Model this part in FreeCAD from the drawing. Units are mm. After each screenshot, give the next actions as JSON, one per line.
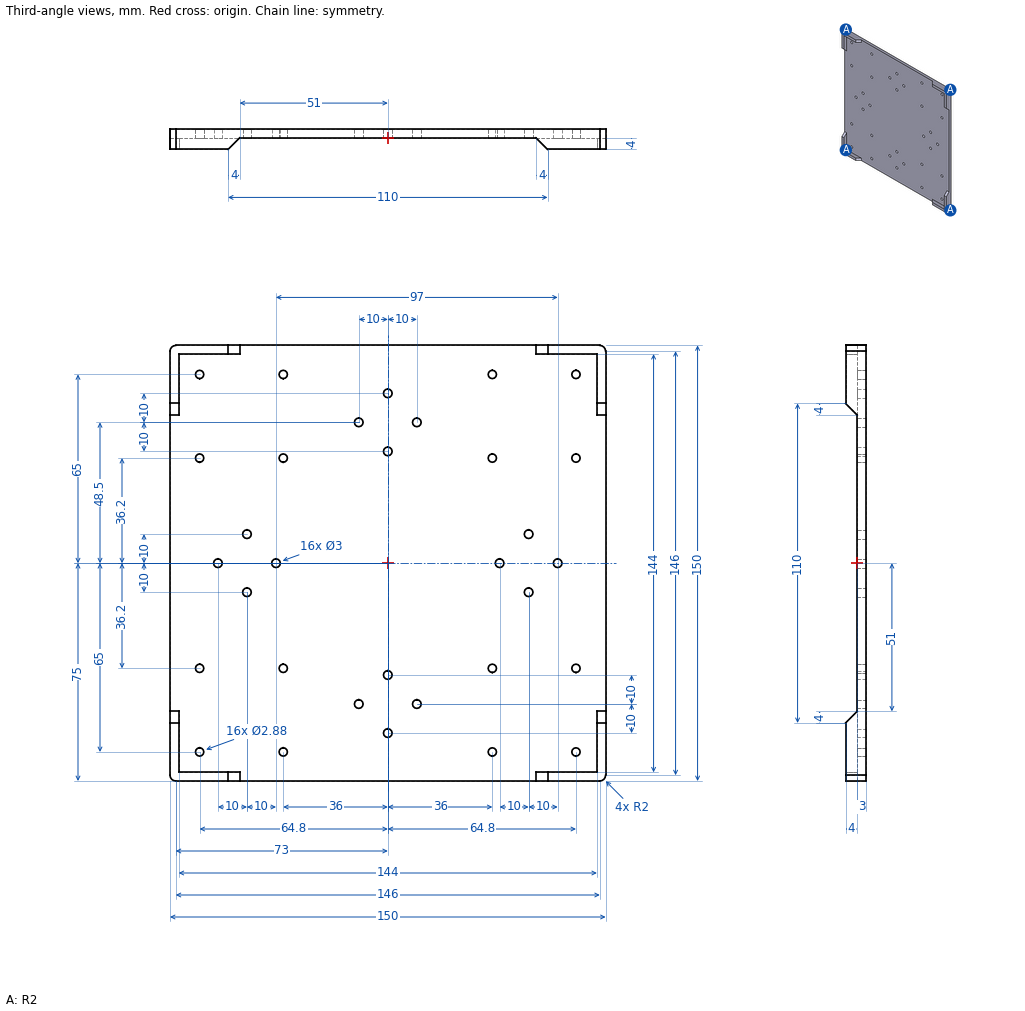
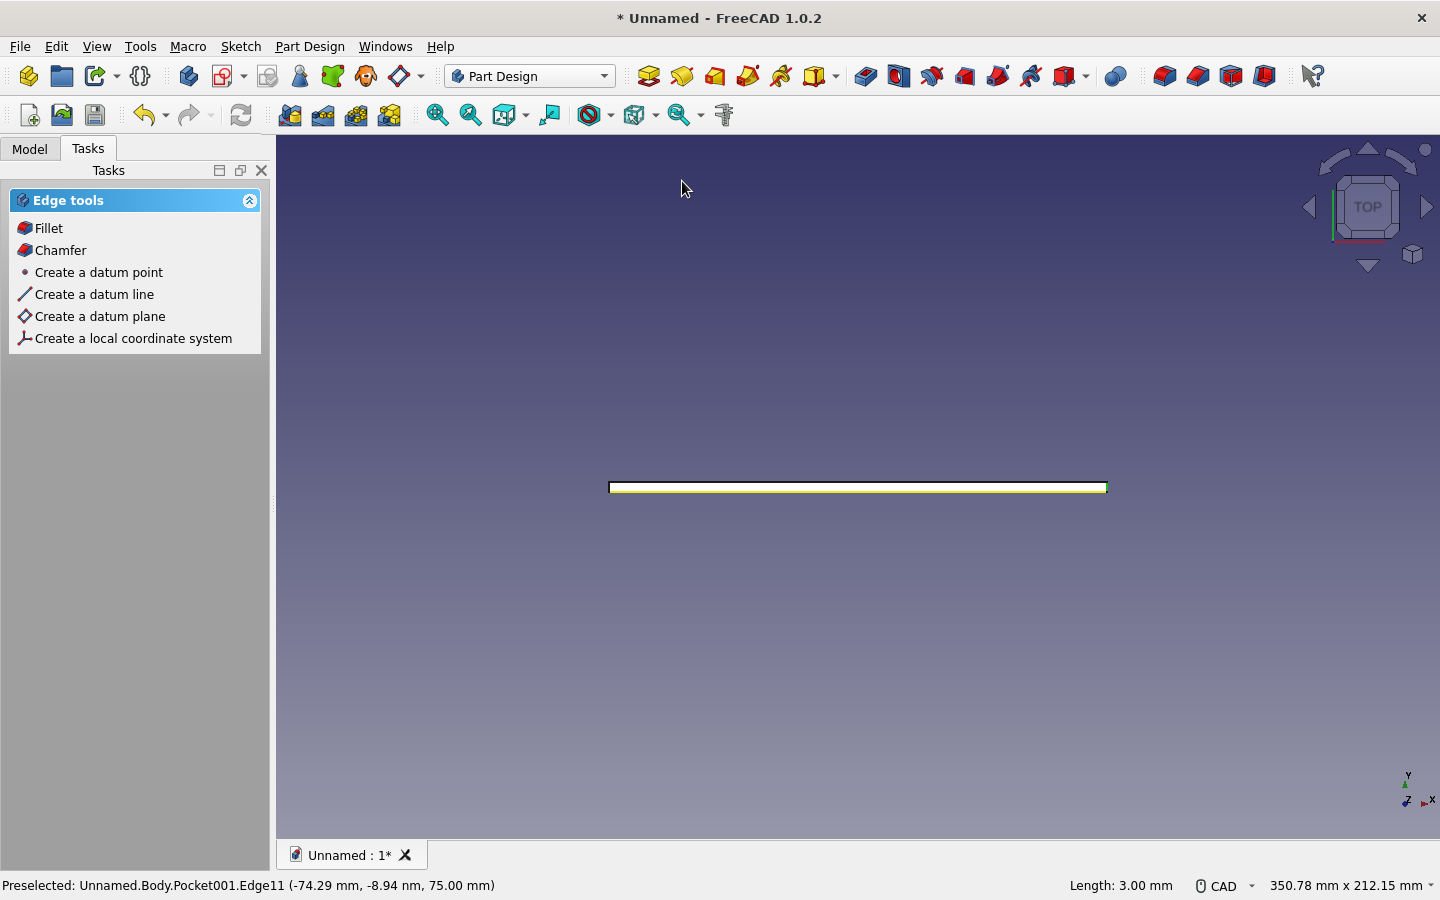
{"action": "left_click", "coordinate": [438, 116]}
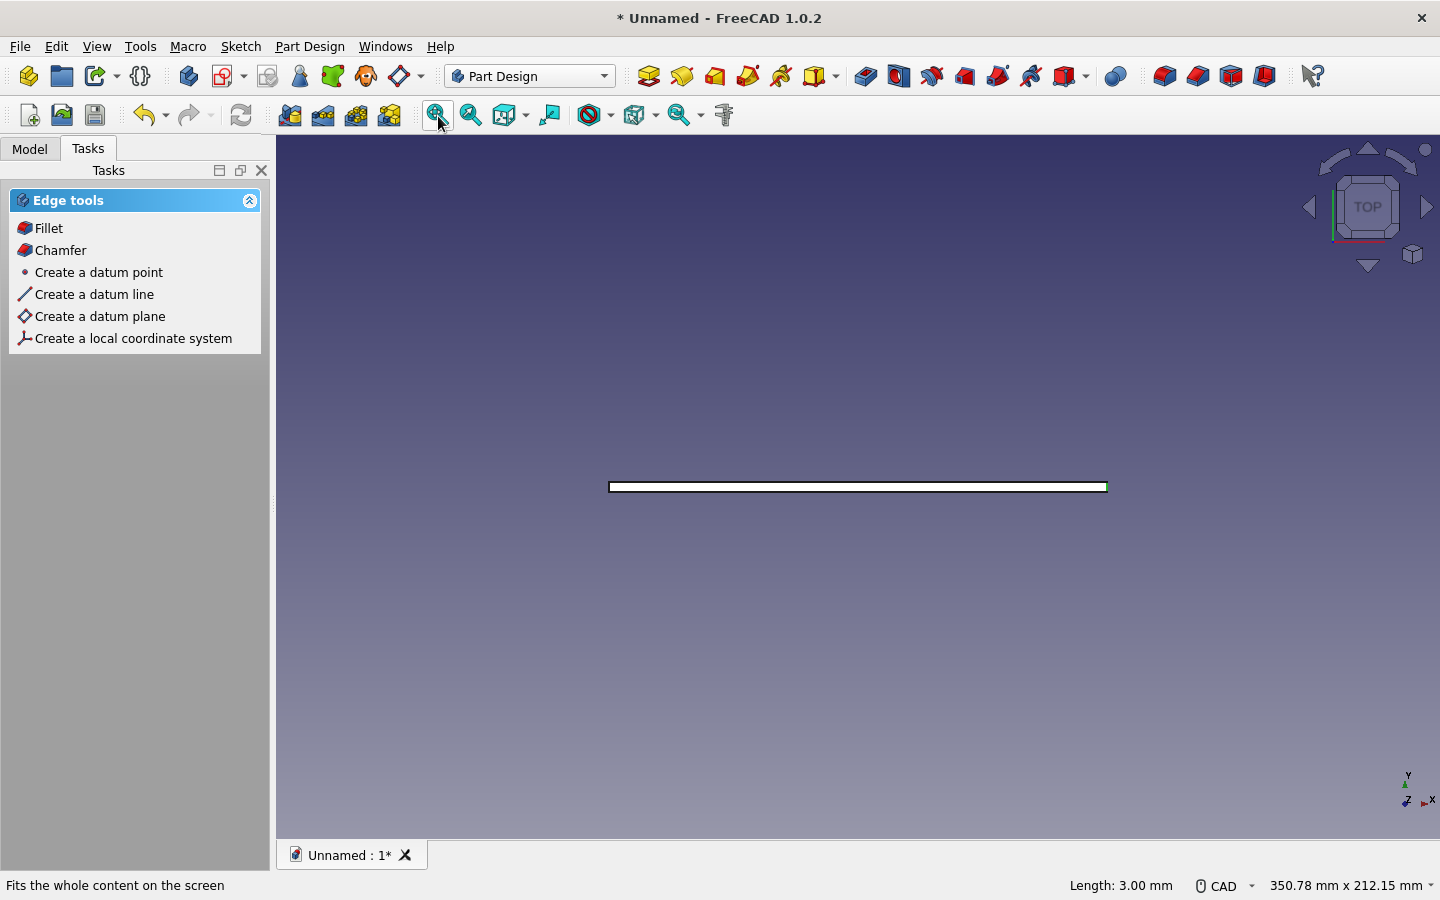
{"action": "left_click", "coordinate": [609, 488], "text": "ctrl"}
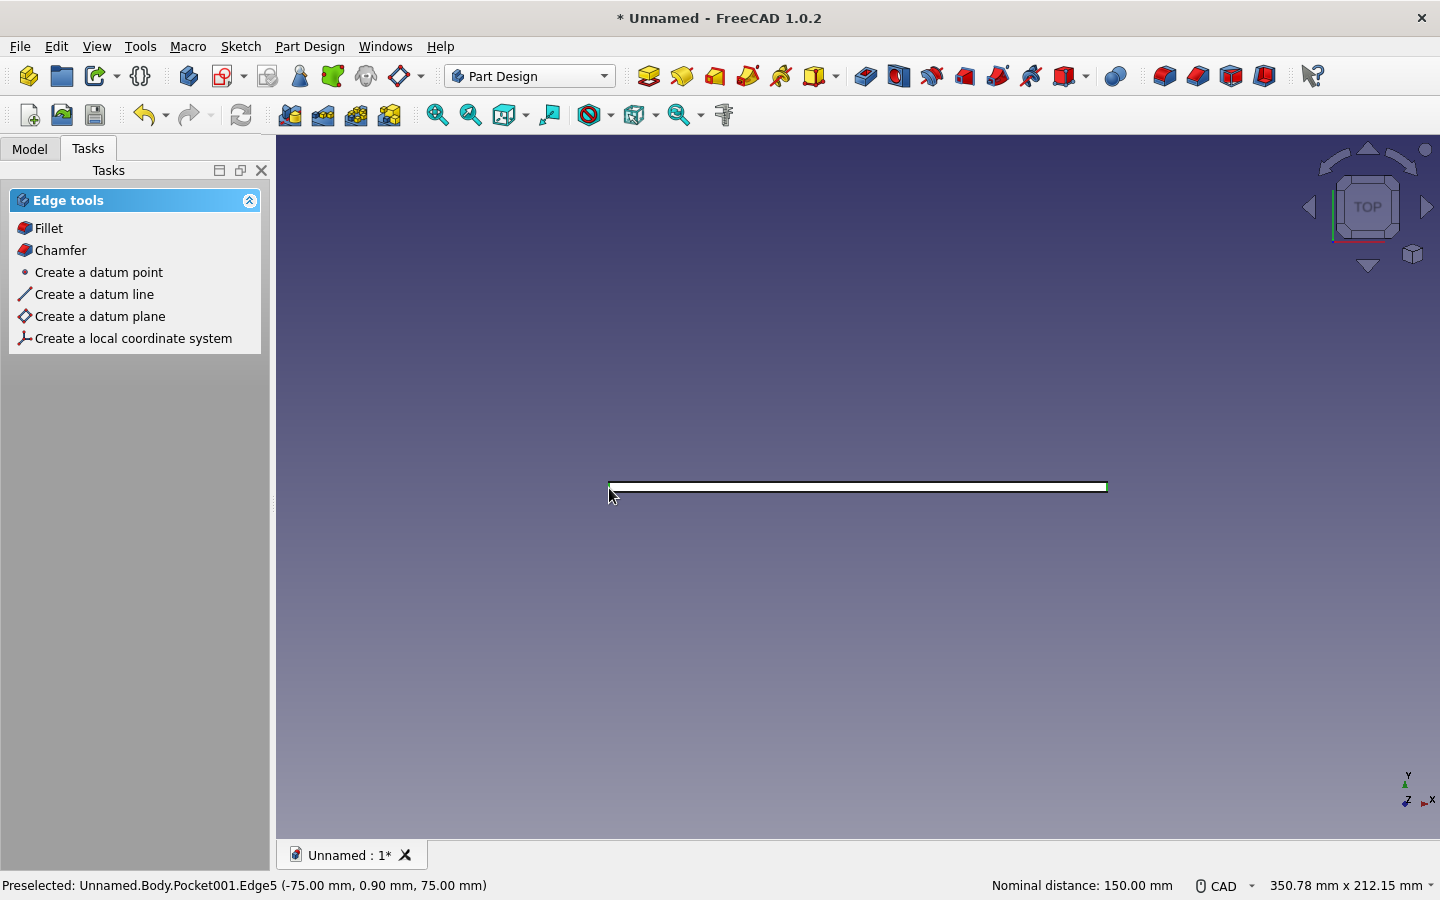
{"action": "scroll", "coordinate": [609, 486], "scroll_direction": "up", "scroll_amount": 7}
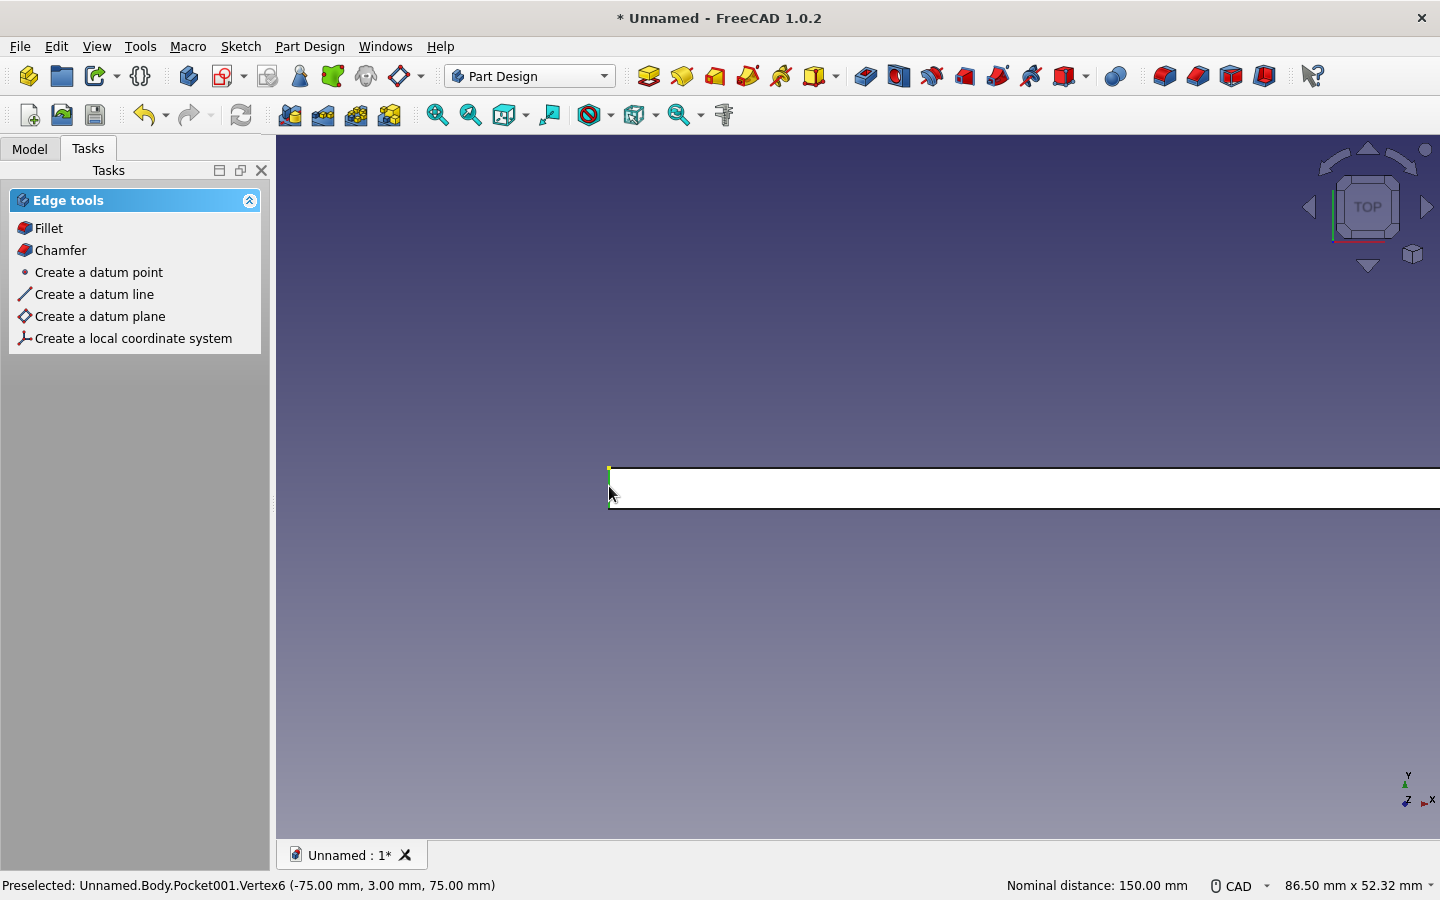
{"action": "left_click", "coordinate": [438, 116]}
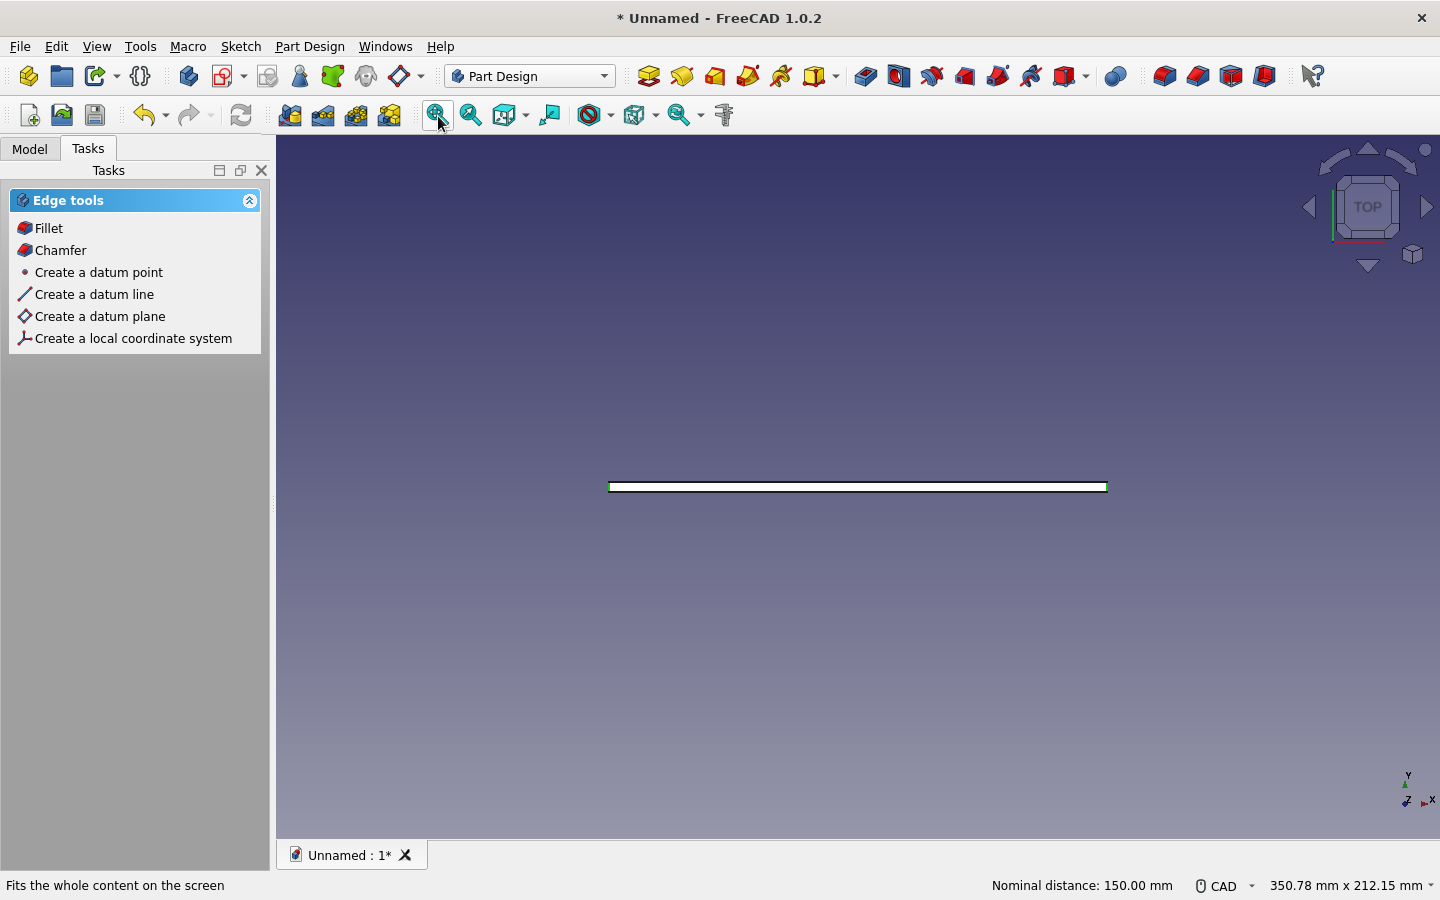
{"action": "key", "text": "1"}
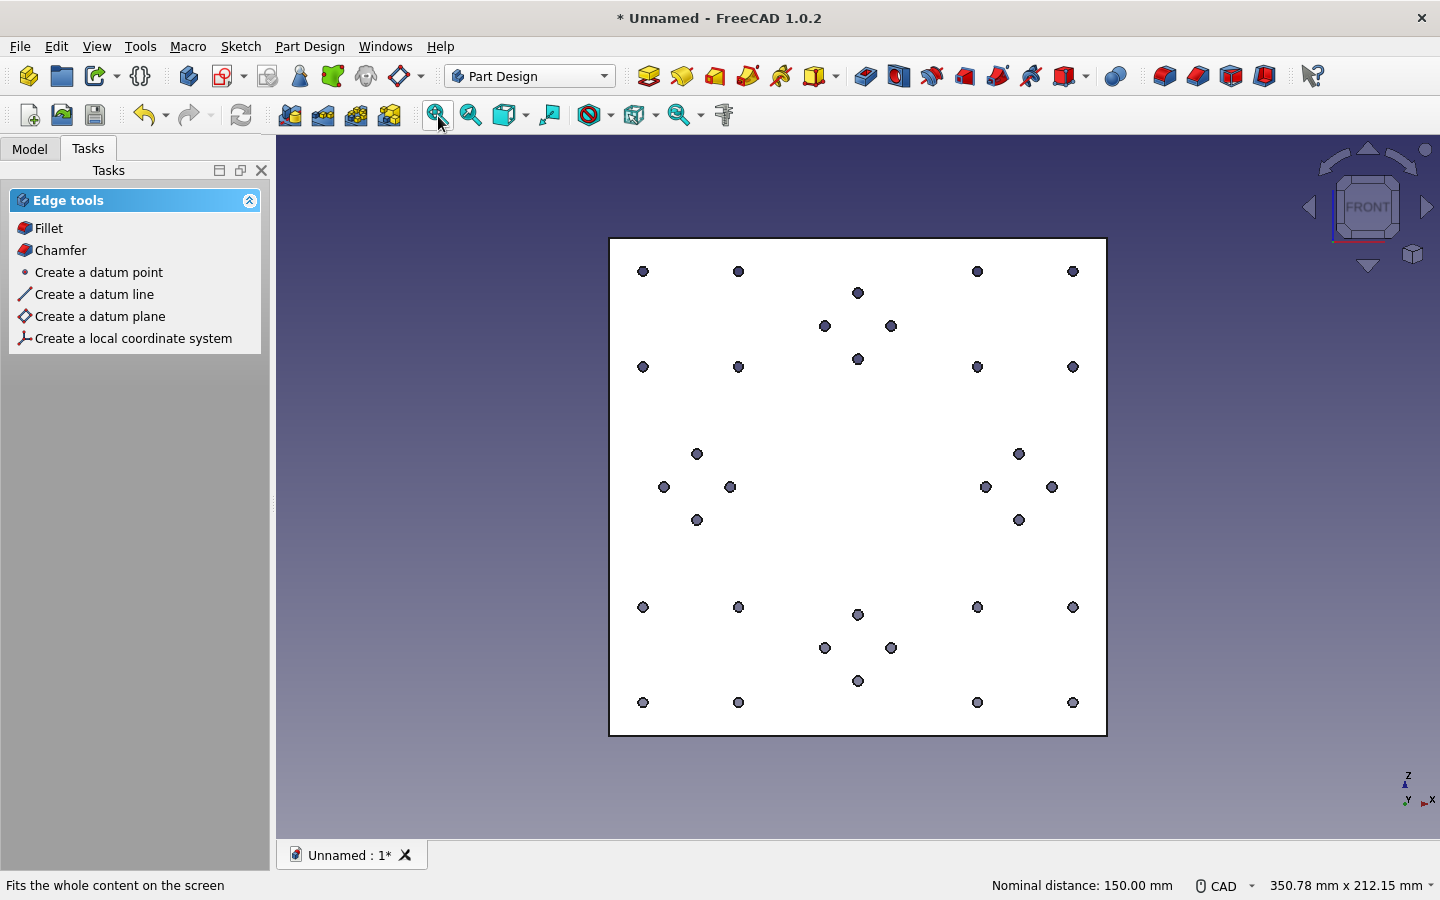
{"action": "scroll", "coordinate": [609, 735], "scroll_direction": "up", "scroll_amount": 7}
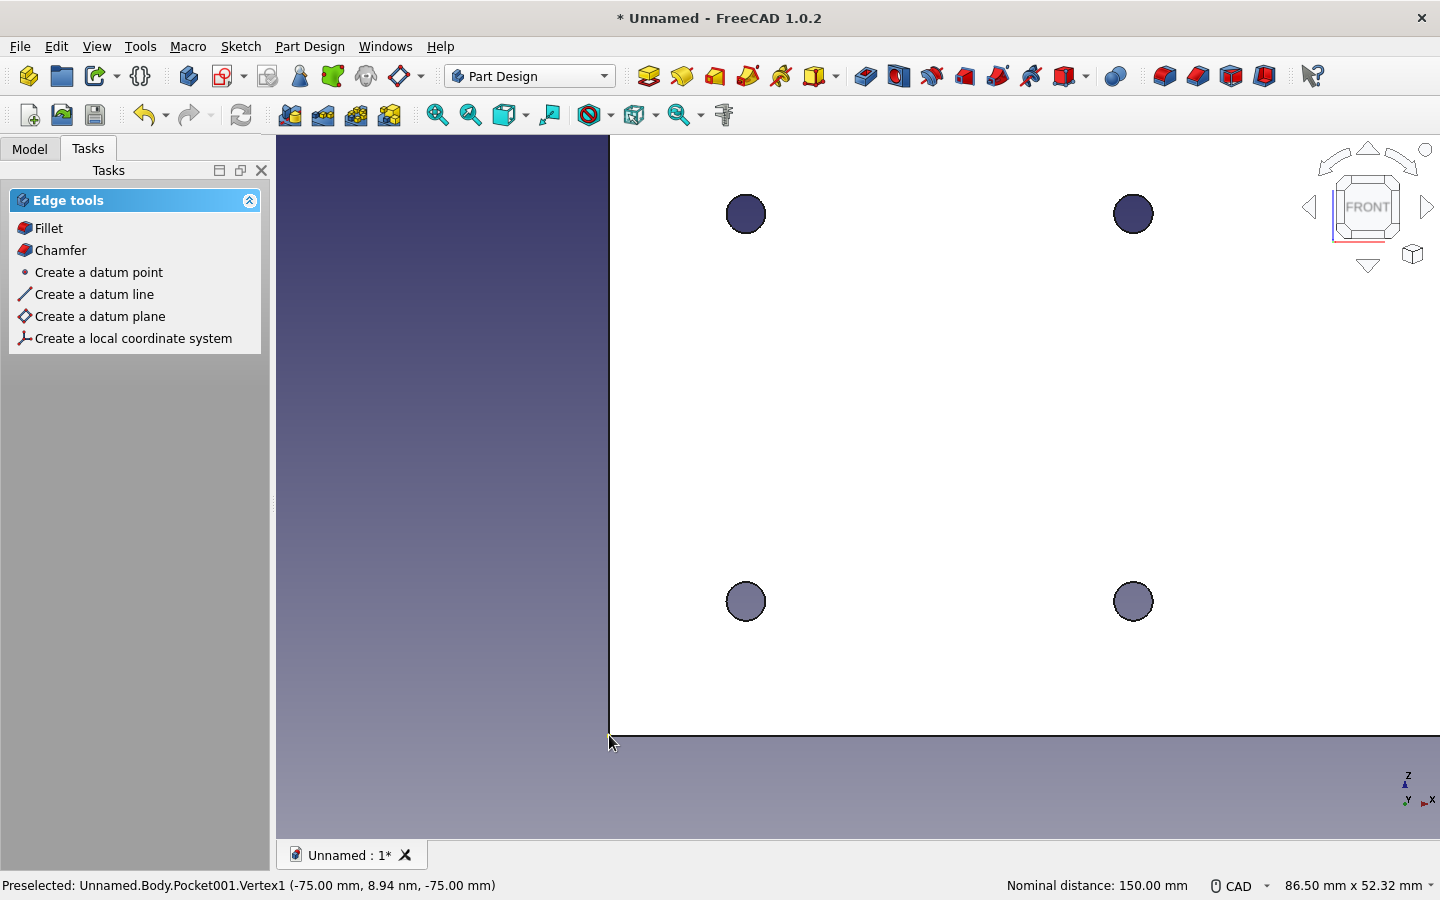
{"action": "left_click", "coordinate": [438, 116]}